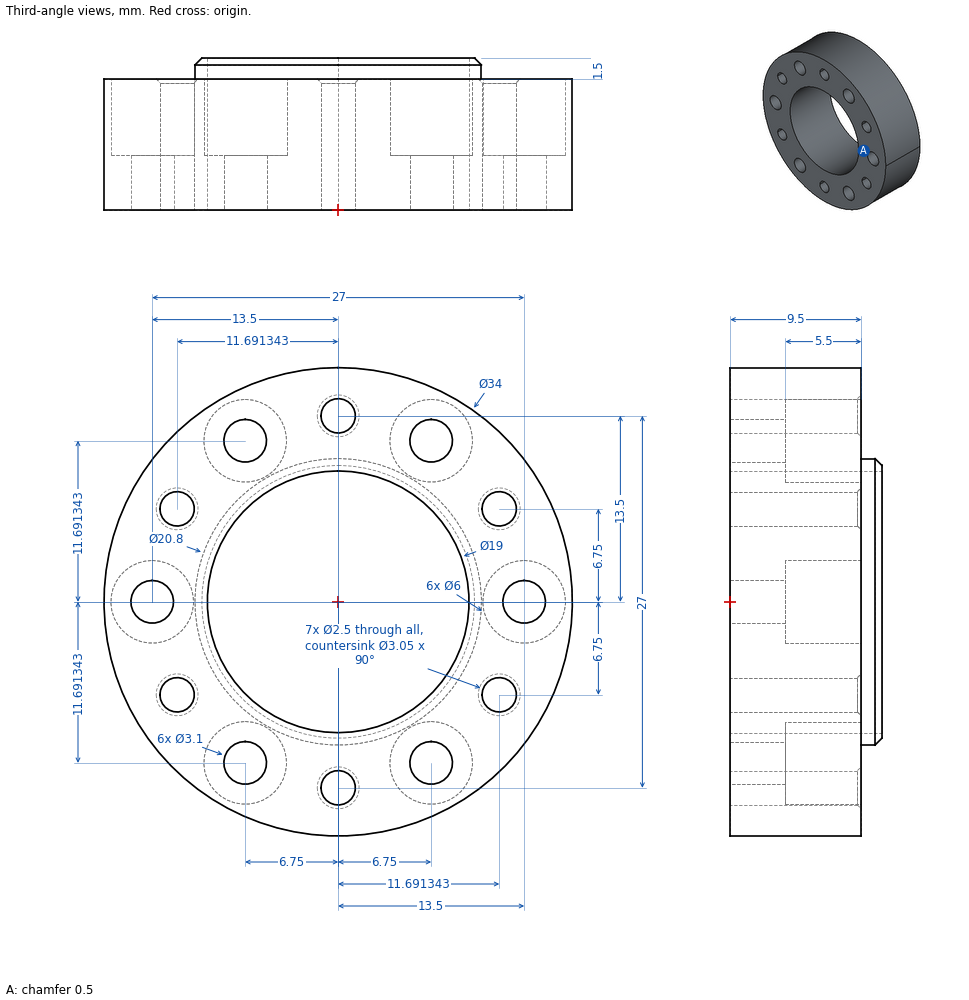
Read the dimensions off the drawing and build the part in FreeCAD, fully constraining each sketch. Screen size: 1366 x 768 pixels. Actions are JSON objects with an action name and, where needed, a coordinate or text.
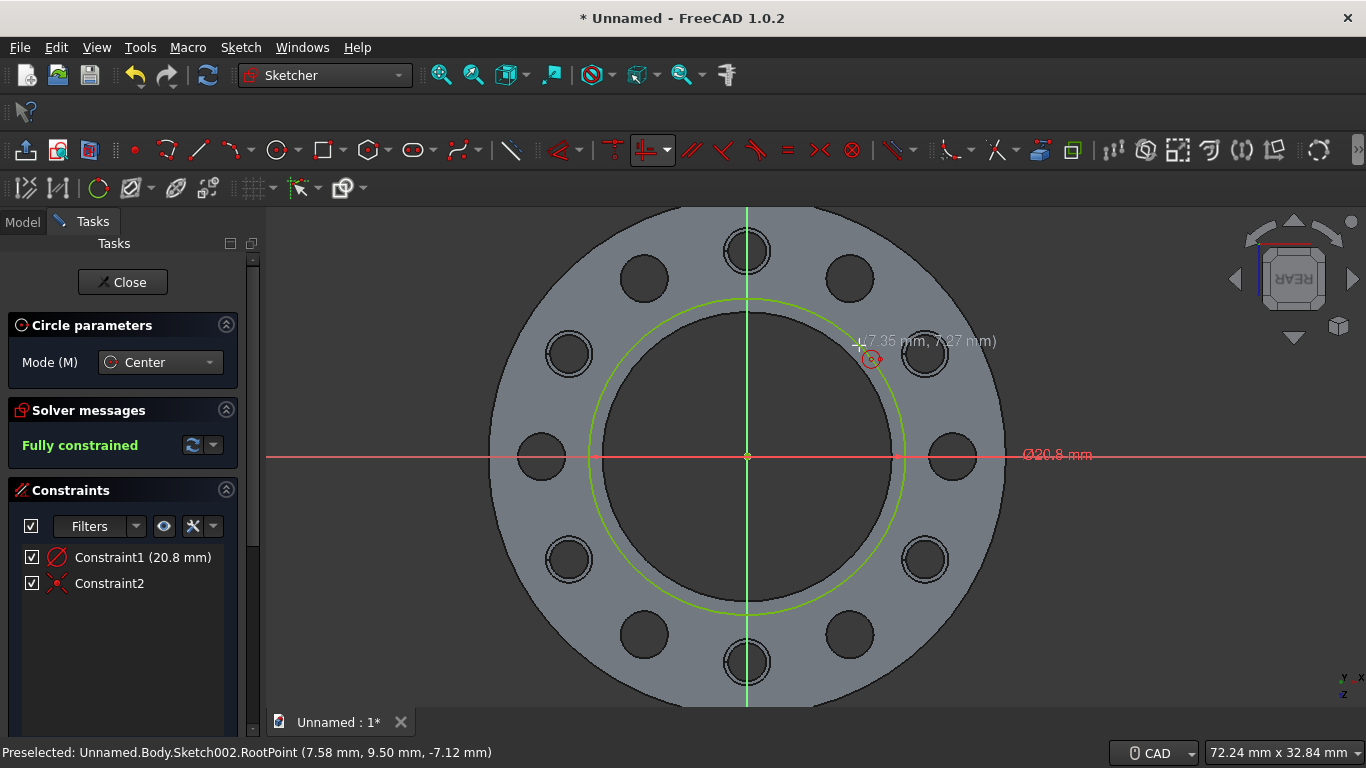
{"action": "left_click", "coordinate": [747, 457]}
{"action": "mouse_move", "coordinate": [849, 354]}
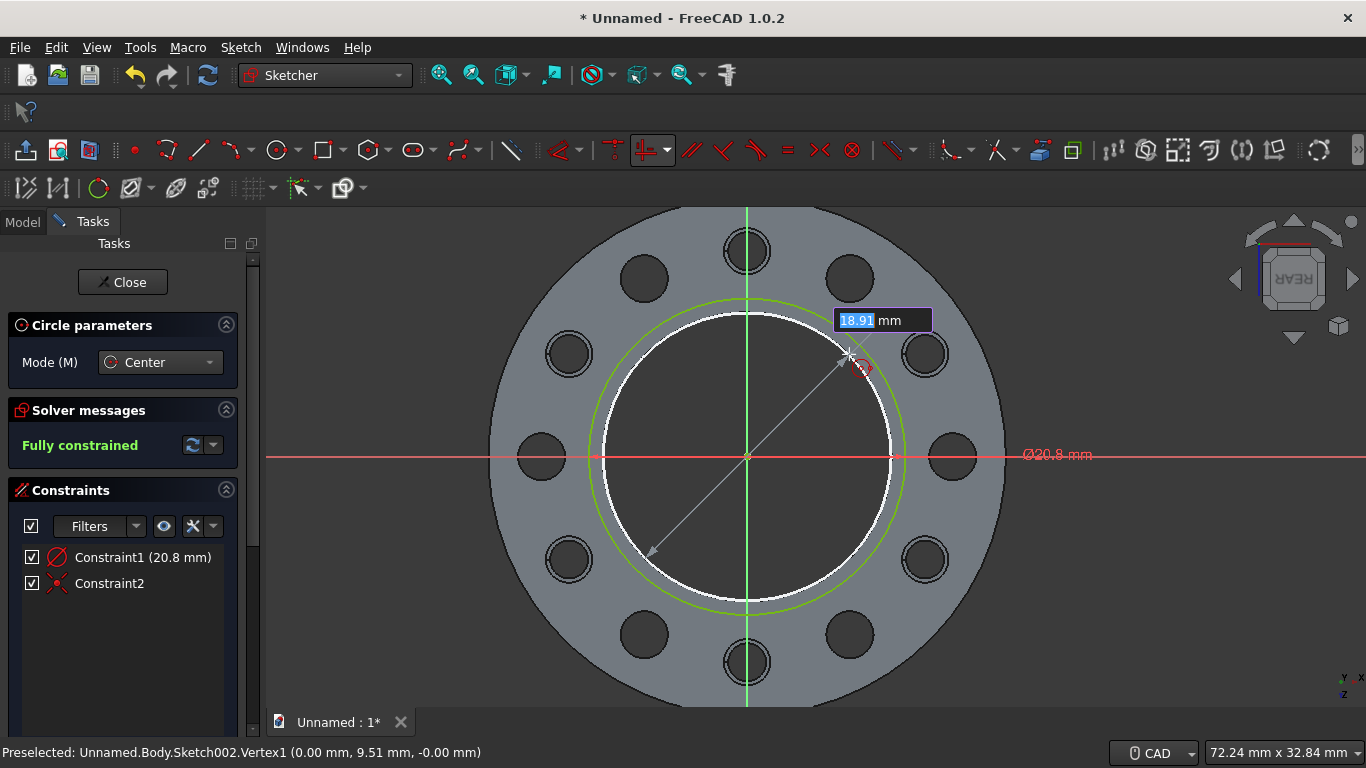
{"action": "type", "text": "19"}
{"action": "key", "text": "Return"}
{"action": "key", "text": "Escape"}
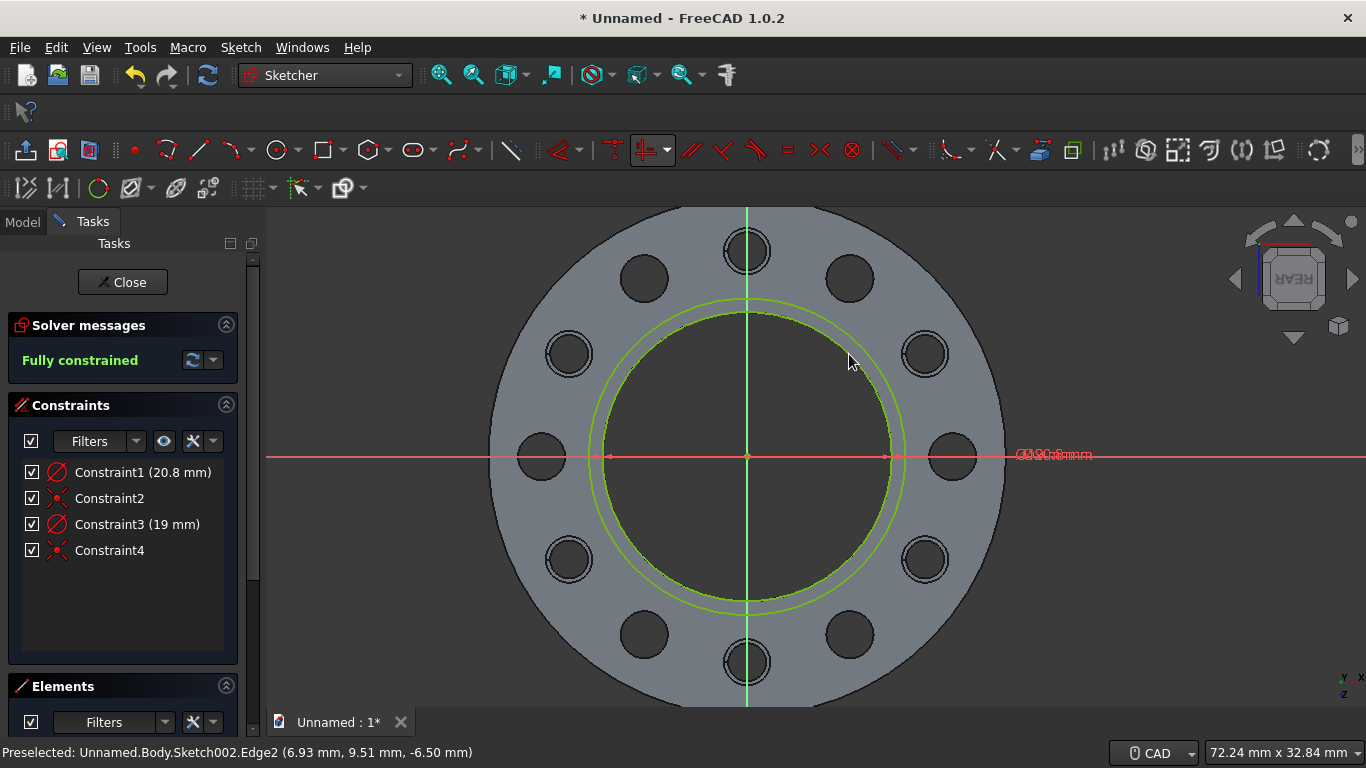
{"action": "left_click", "coordinate": [123, 282]}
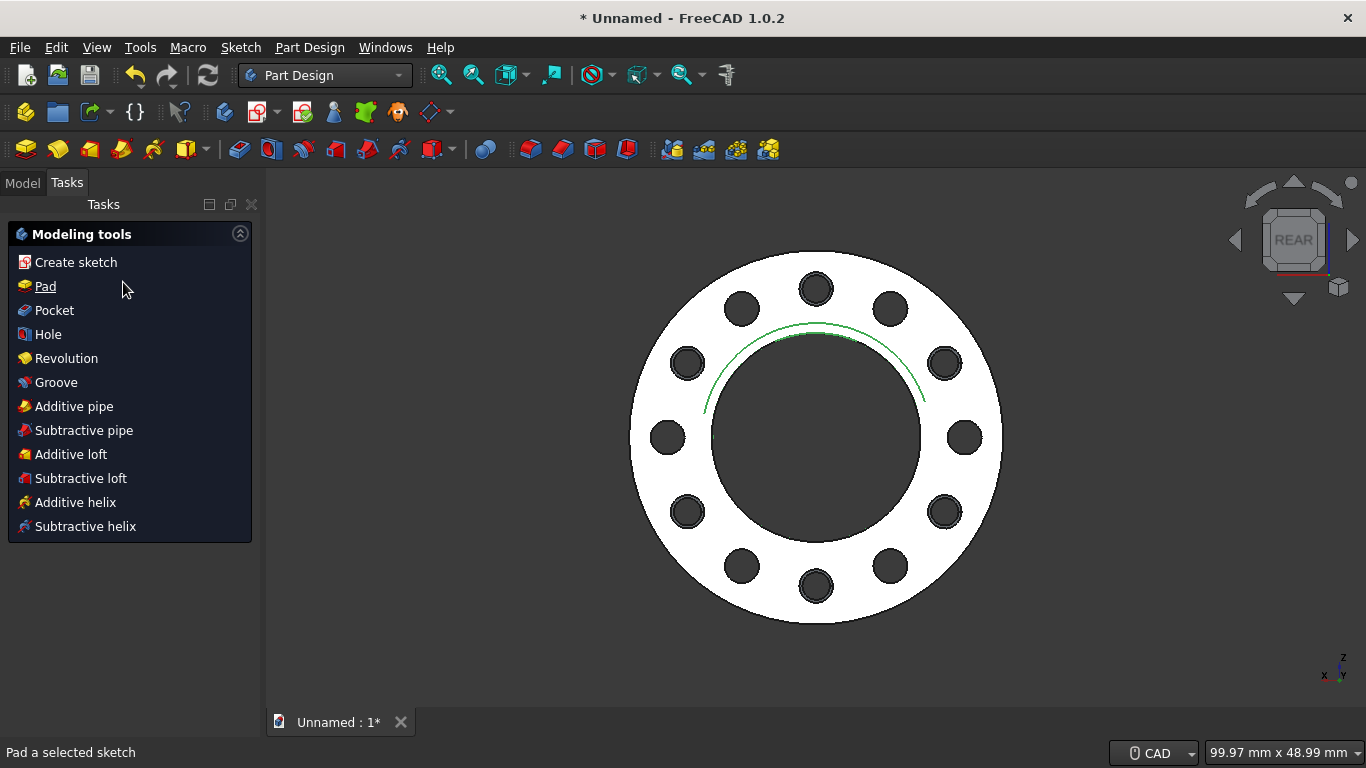
{"action": "left_click", "coordinate": [26, 150]}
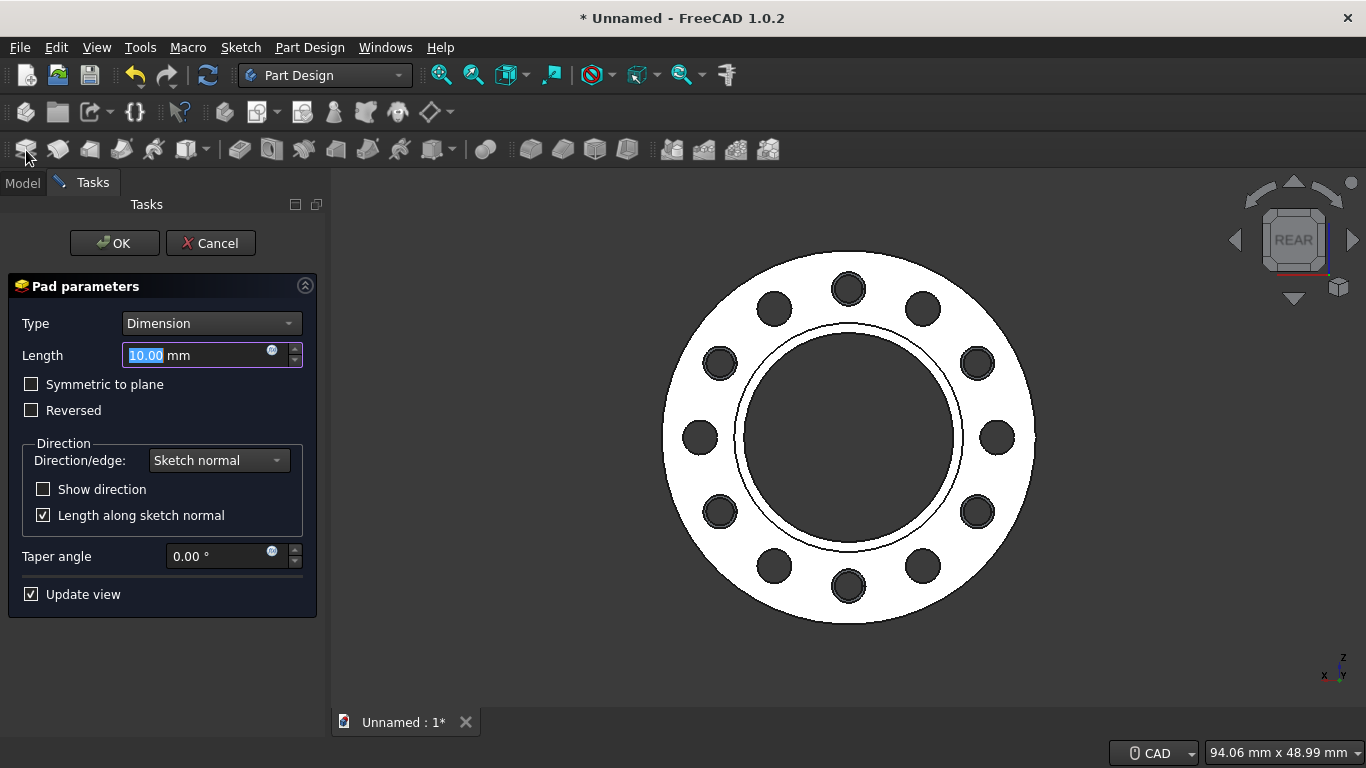
{"action": "type", "text": "1.5"}
{"action": "key", "text": "Tab"}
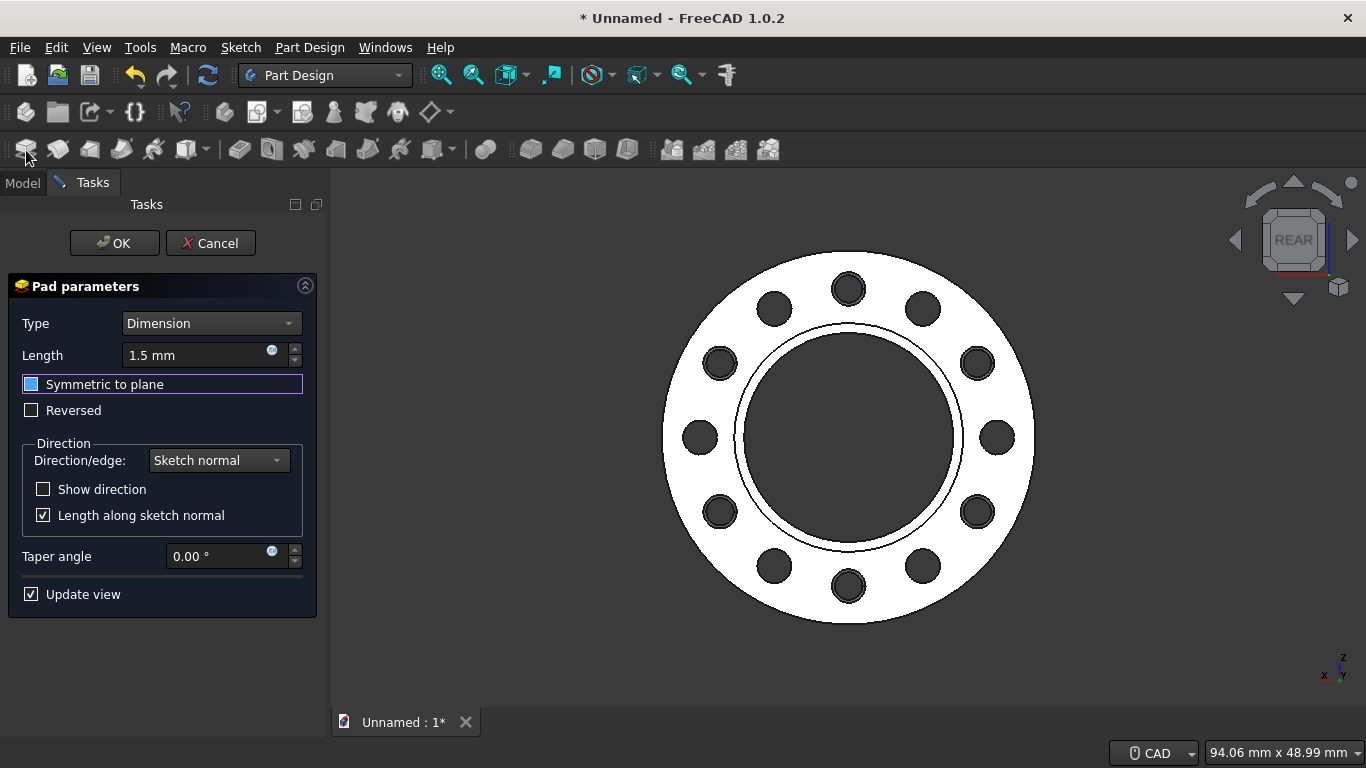
{"action": "left_click", "coordinate": [115, 243]}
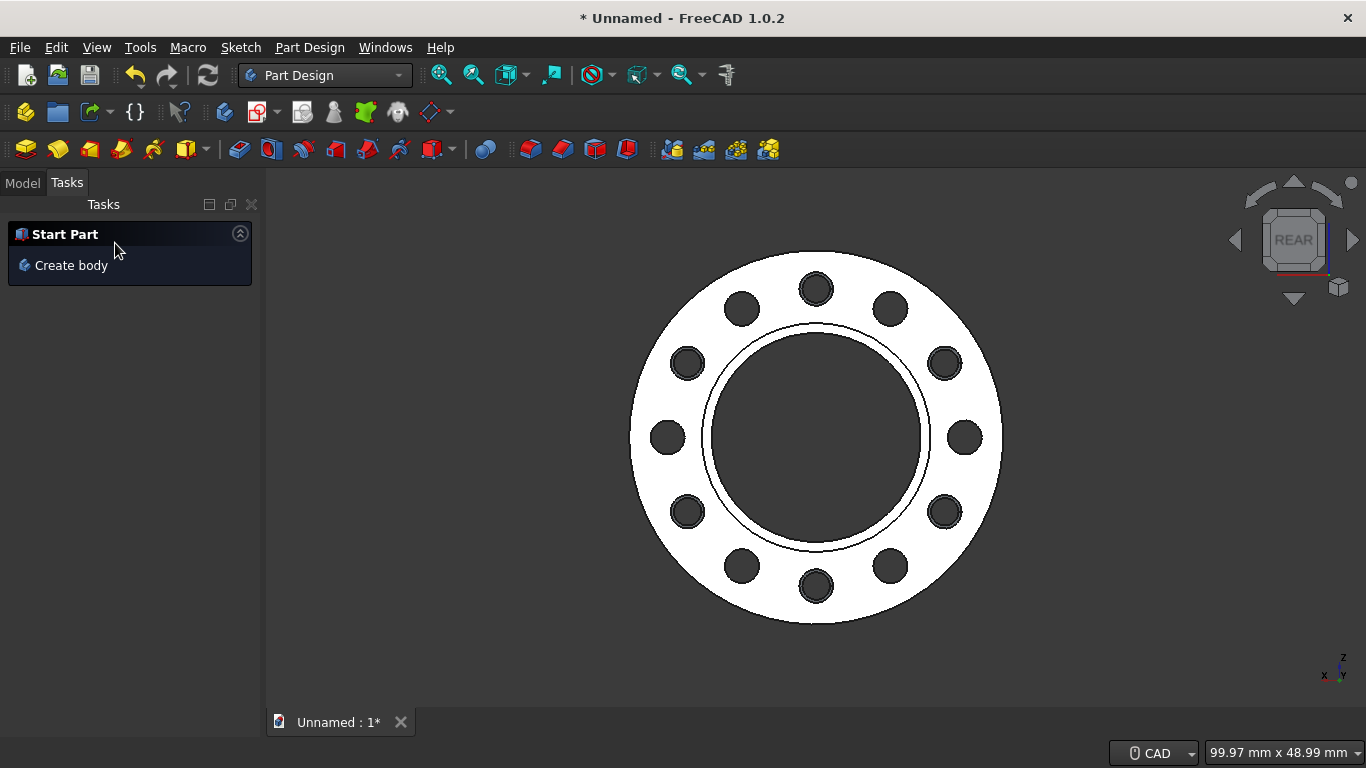
{"action": "left_click", "coordinate": [709, 330]}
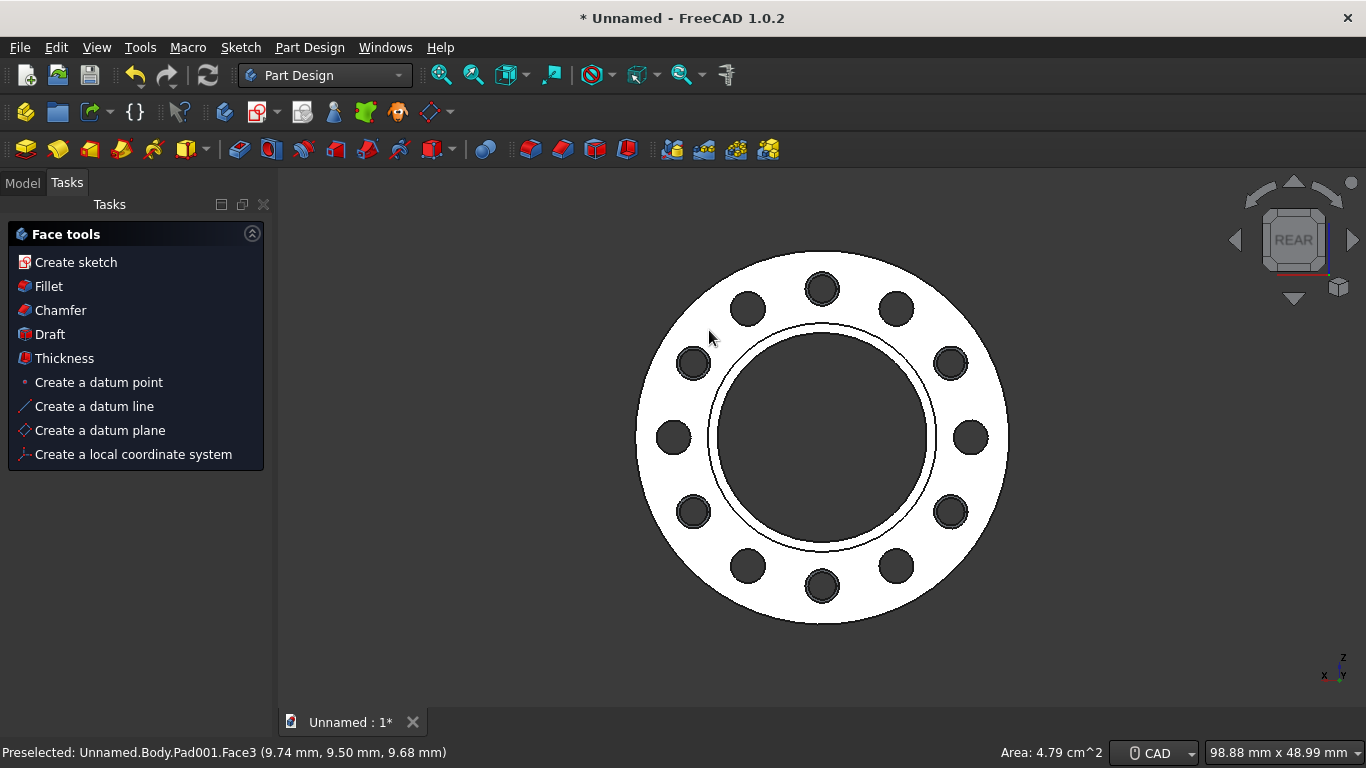
{"action": "left_click", "coordinate": [258, 112]}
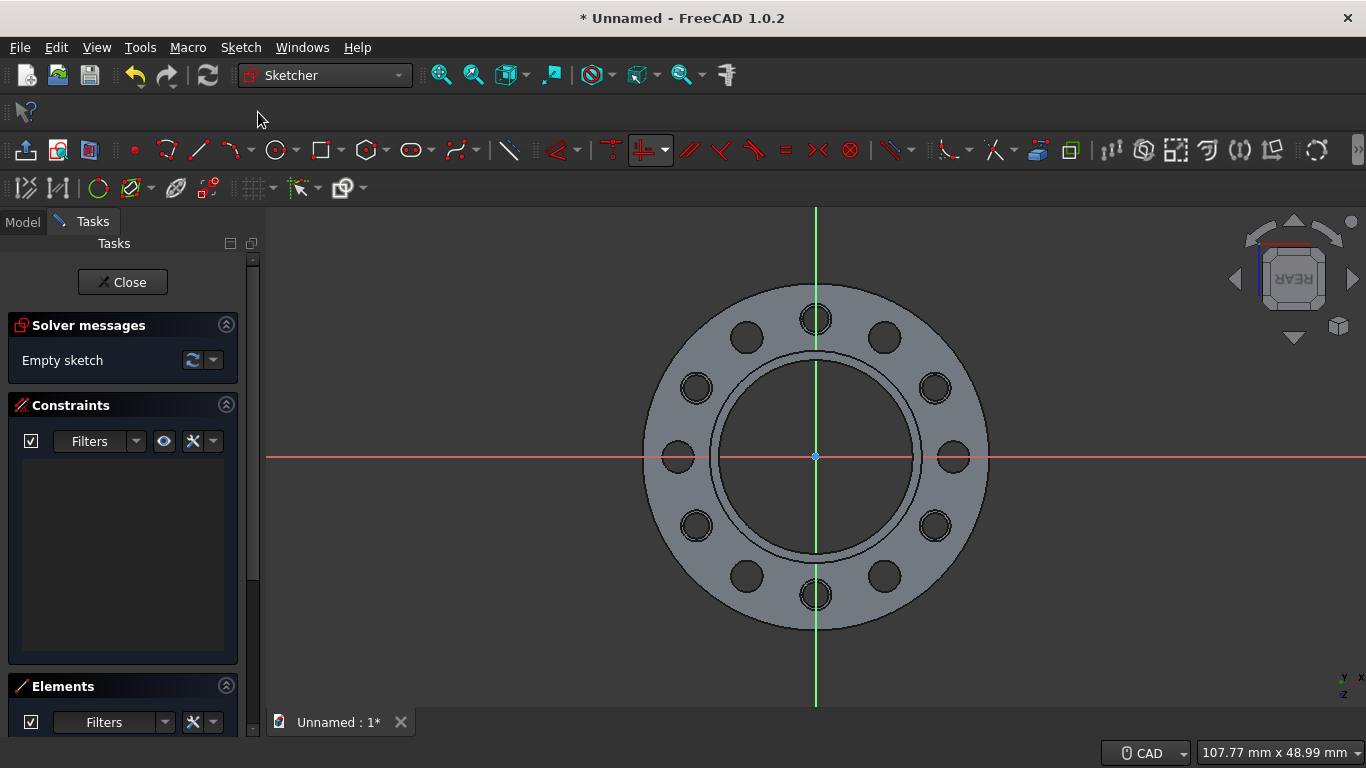
{"action": "left_click", "coordinate": [276, 150]}